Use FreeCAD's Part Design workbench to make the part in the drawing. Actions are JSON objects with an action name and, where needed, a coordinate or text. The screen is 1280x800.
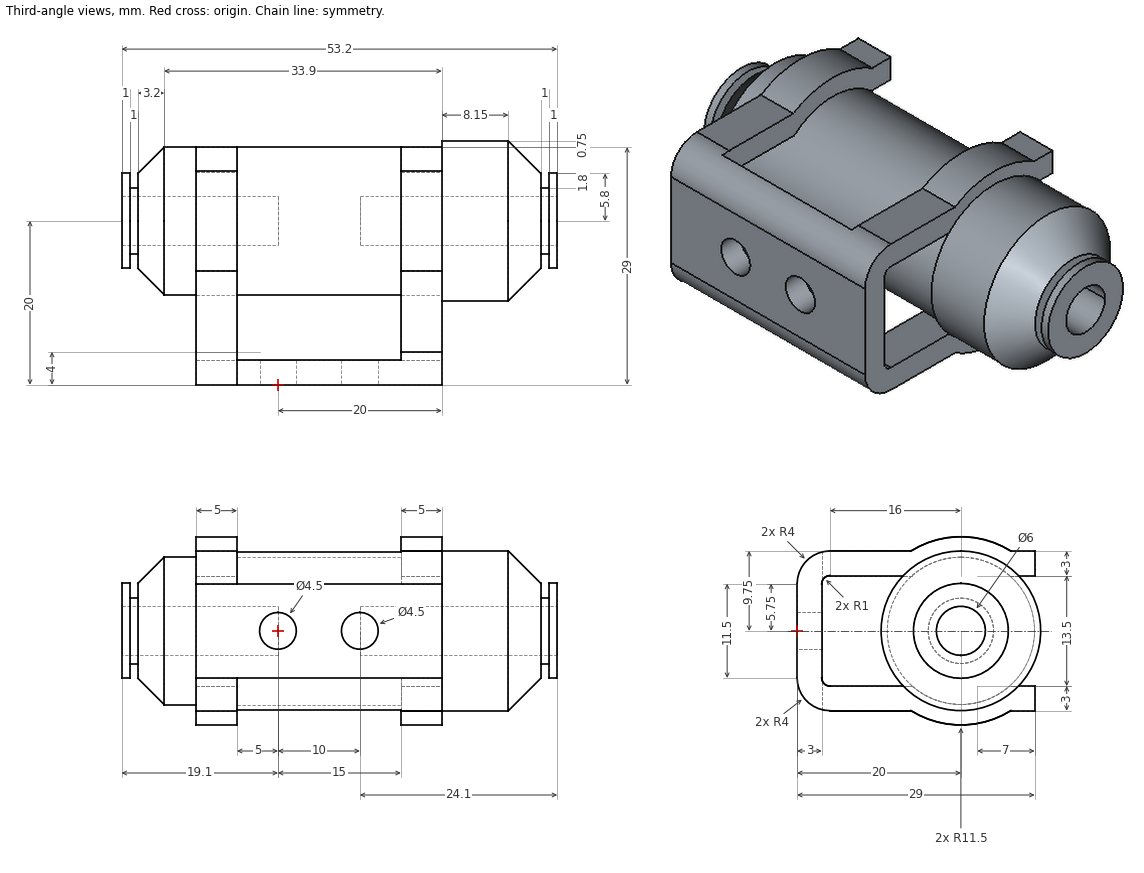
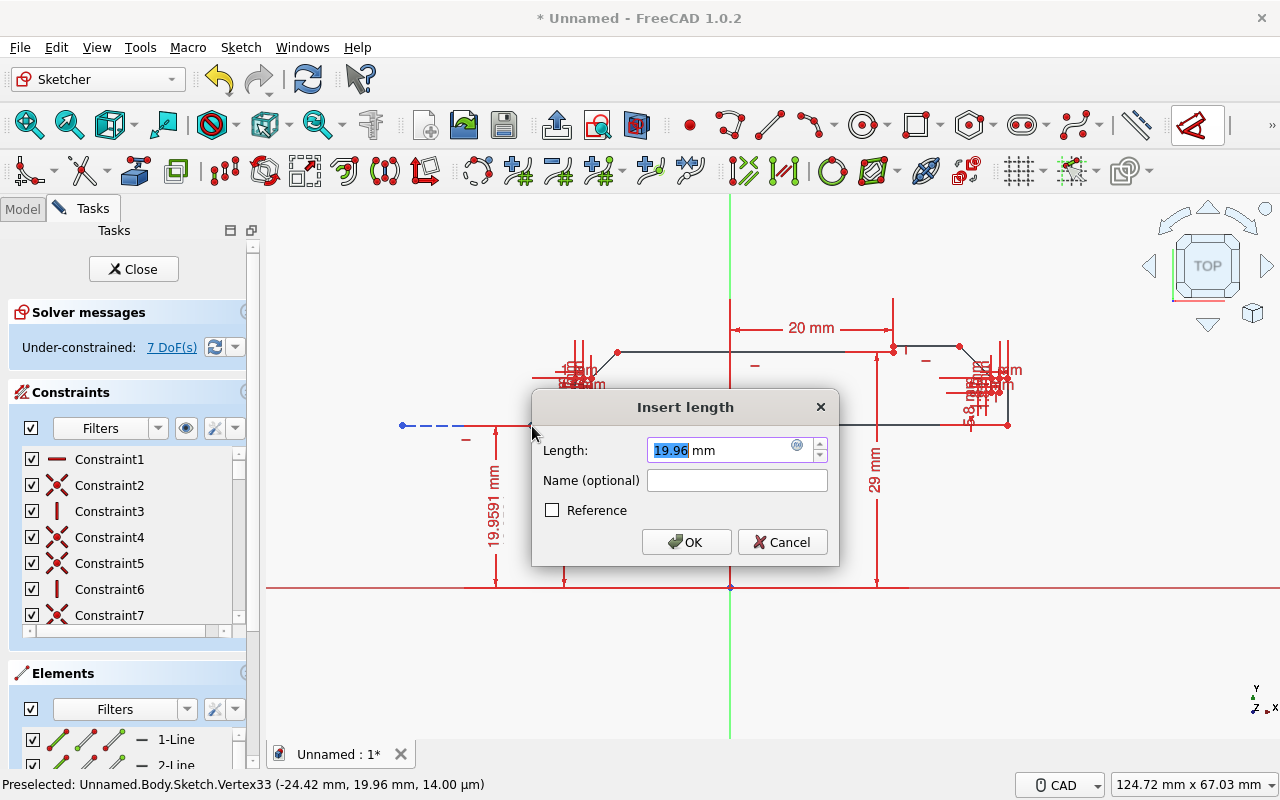
{"action": "type", "text": "20"}
{"action": "key", "text": "Return"}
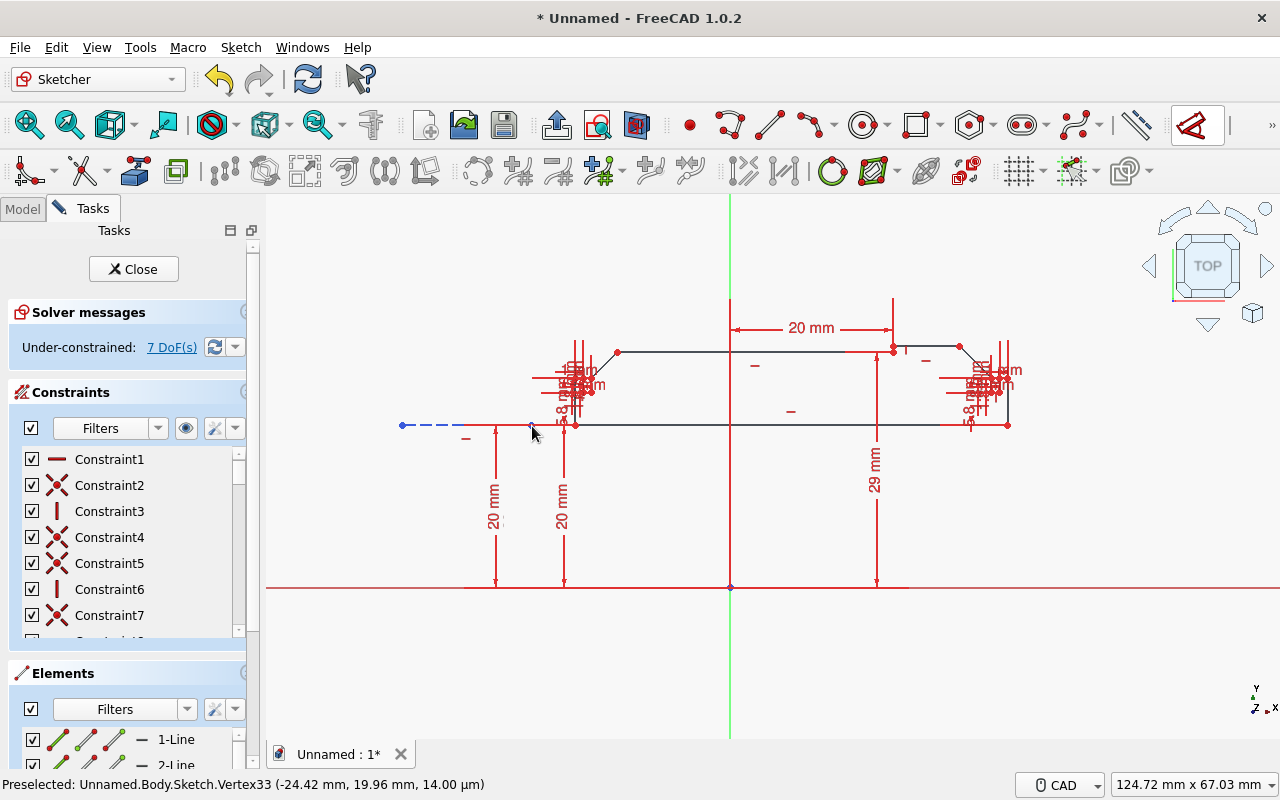
{"action": "left_click", "coordinate": [705, 425]}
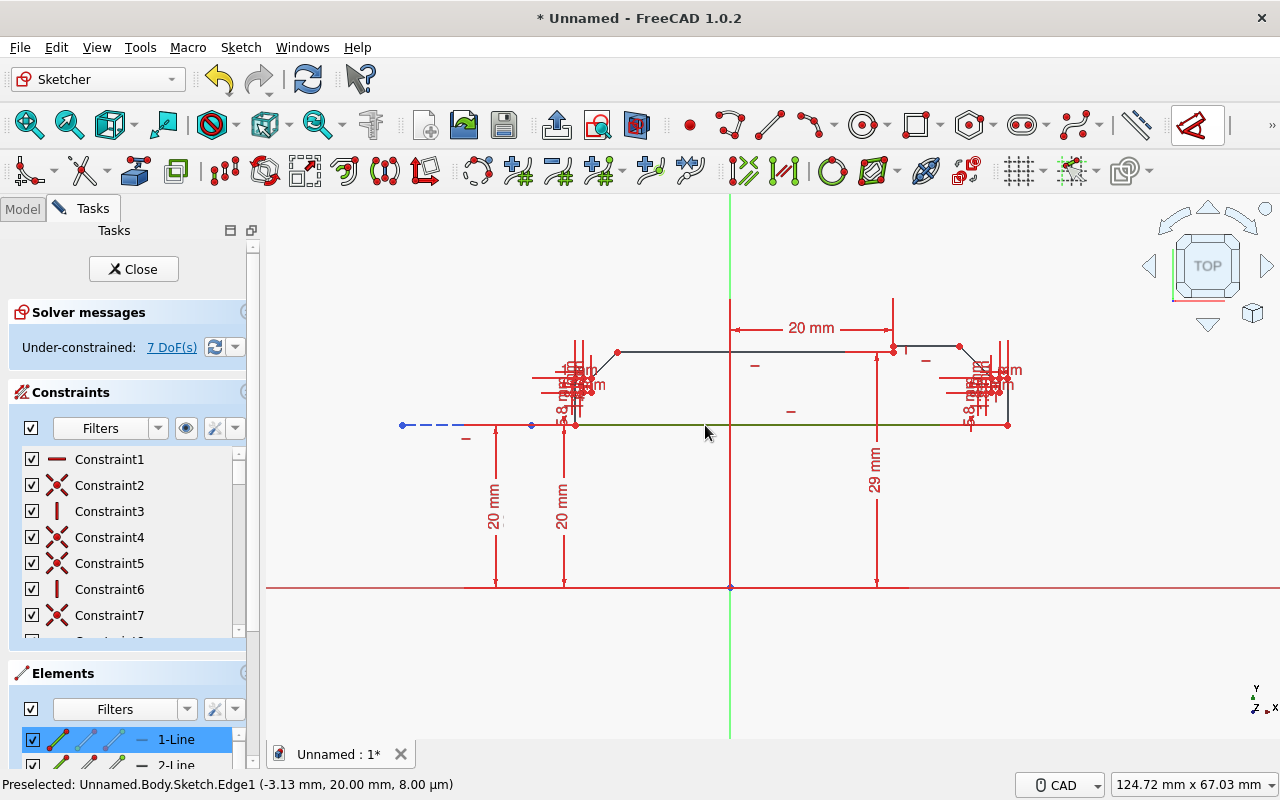
{"action": "left_click", "coordinate": [1218, 126]}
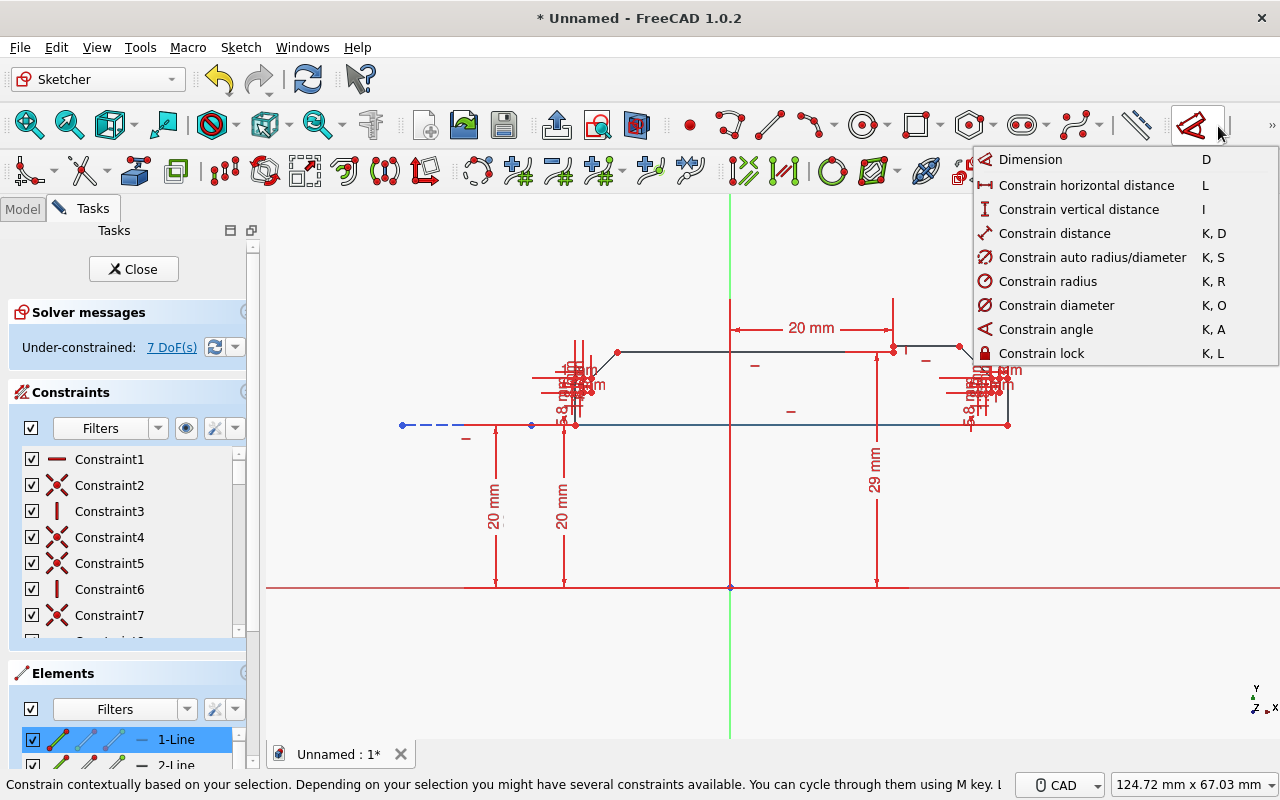
{"action": "left_click", "coordinate": [1126, 185]}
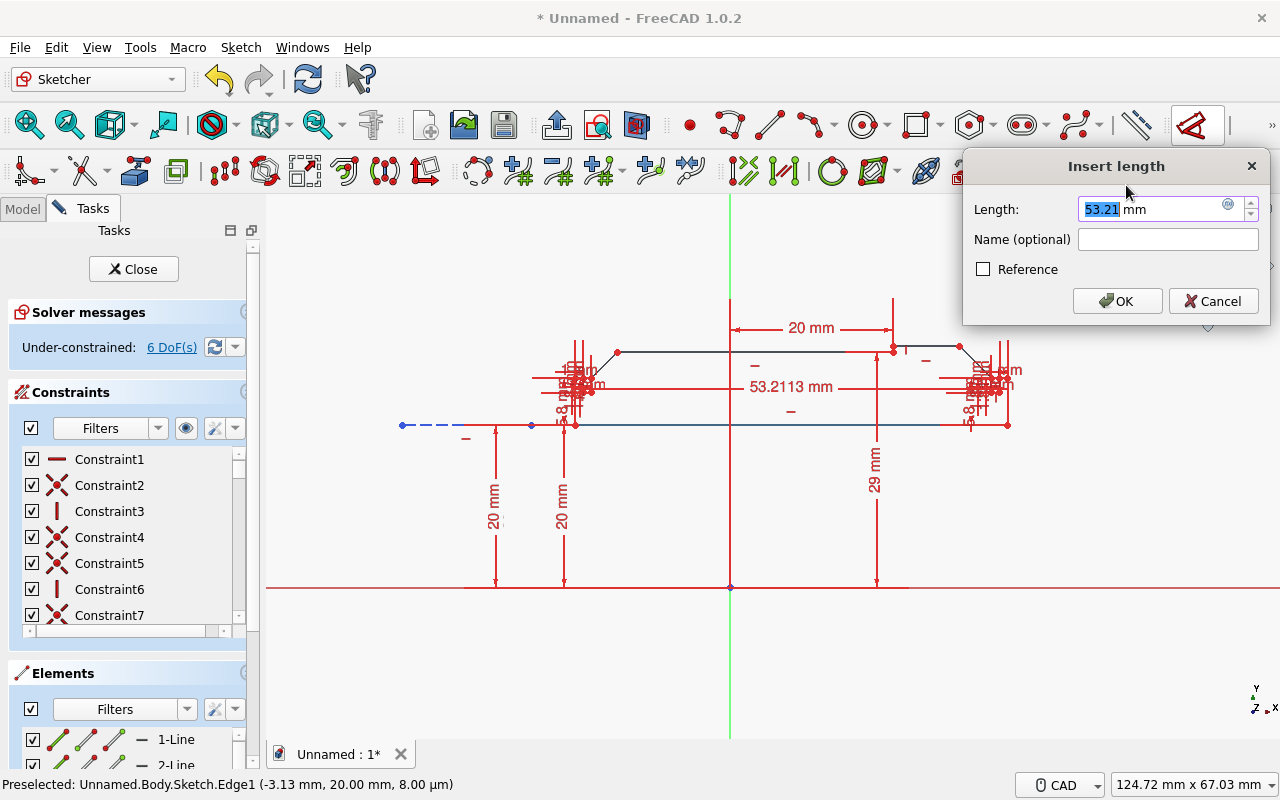
{"action": "type", "text": "53.2"}
{"action": "key", "text": "Return"}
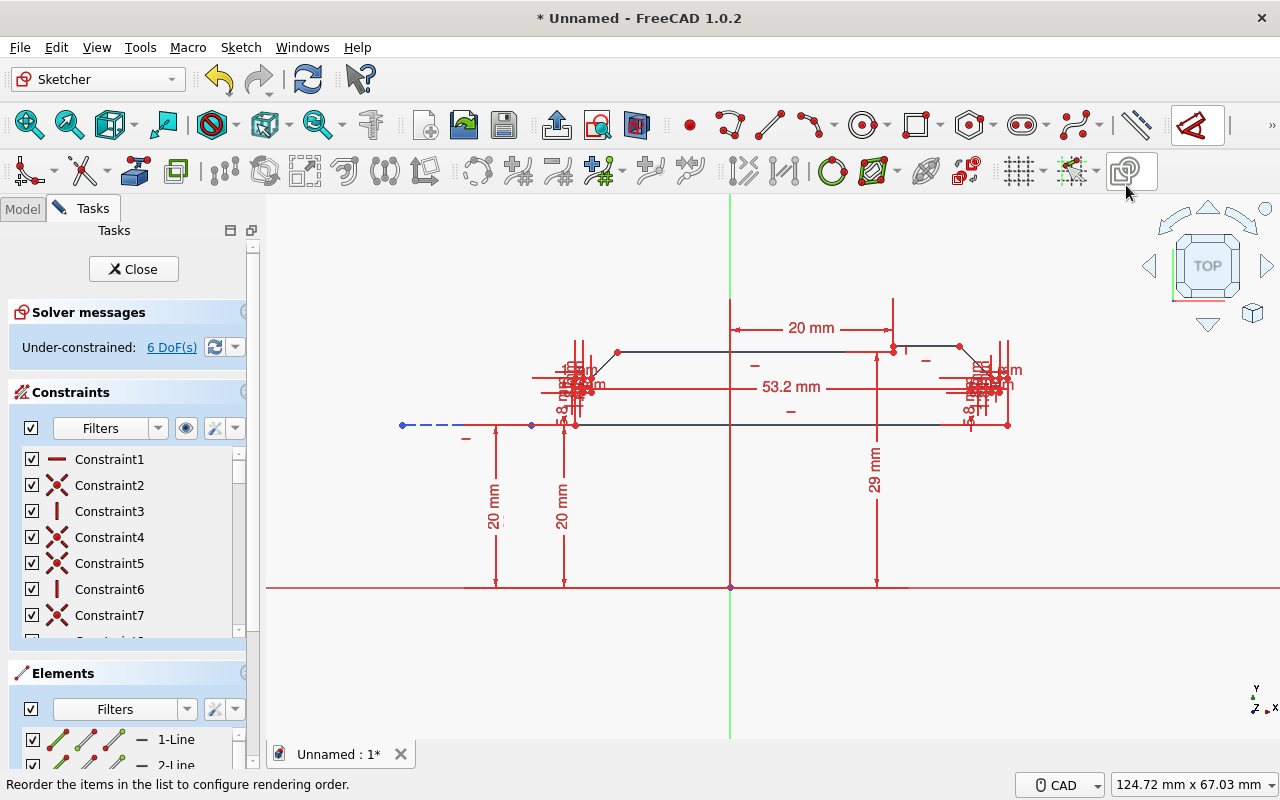
{"action": "left_click", "coordinate": [940, 346]}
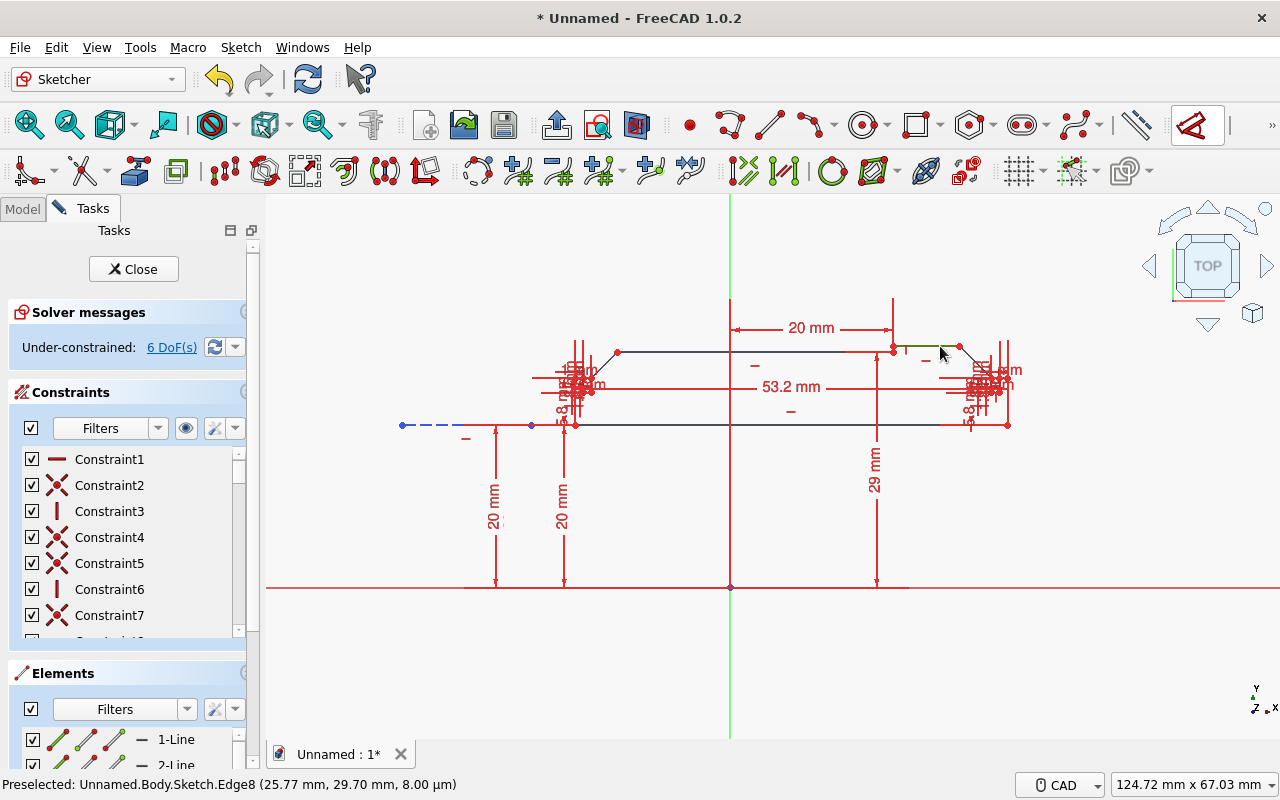
{"action": "key", "text": "l"}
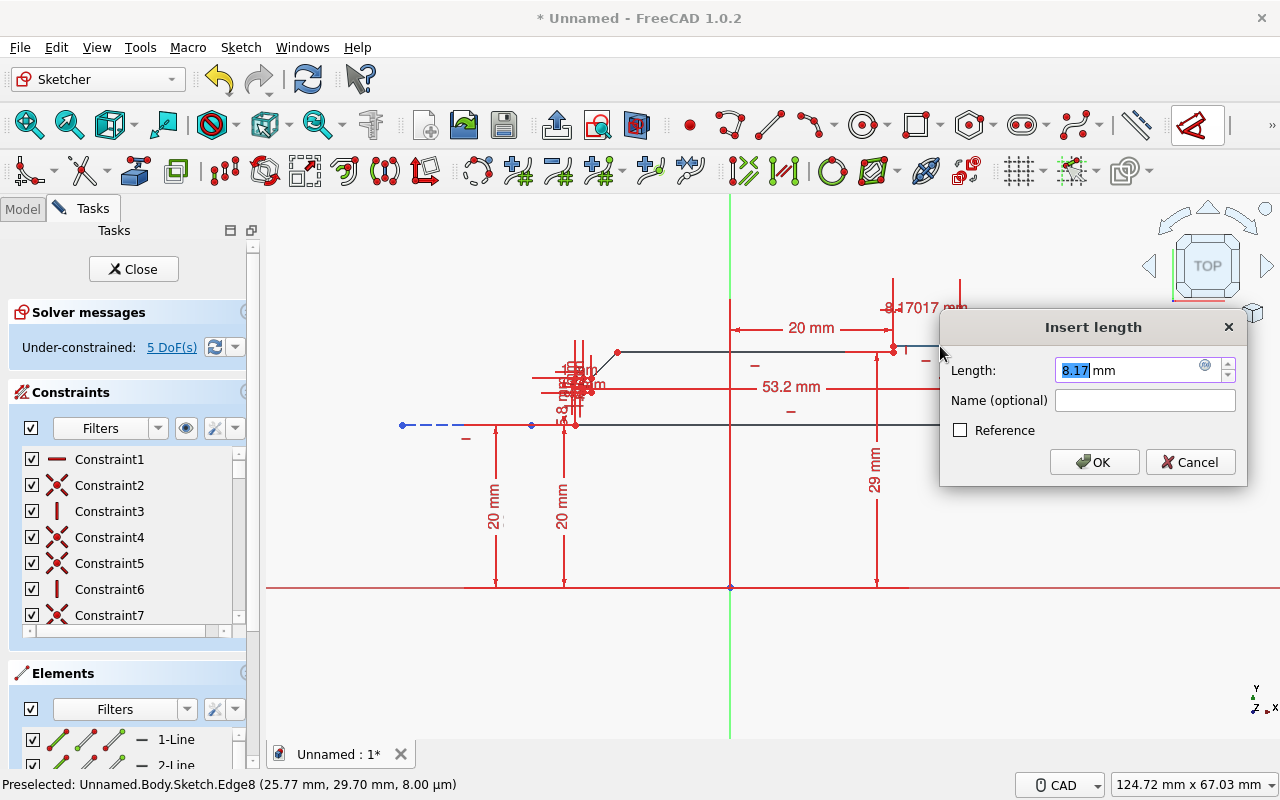
{"action": "type", "text": "8.15"}
{"action": "key", "text": "Return"}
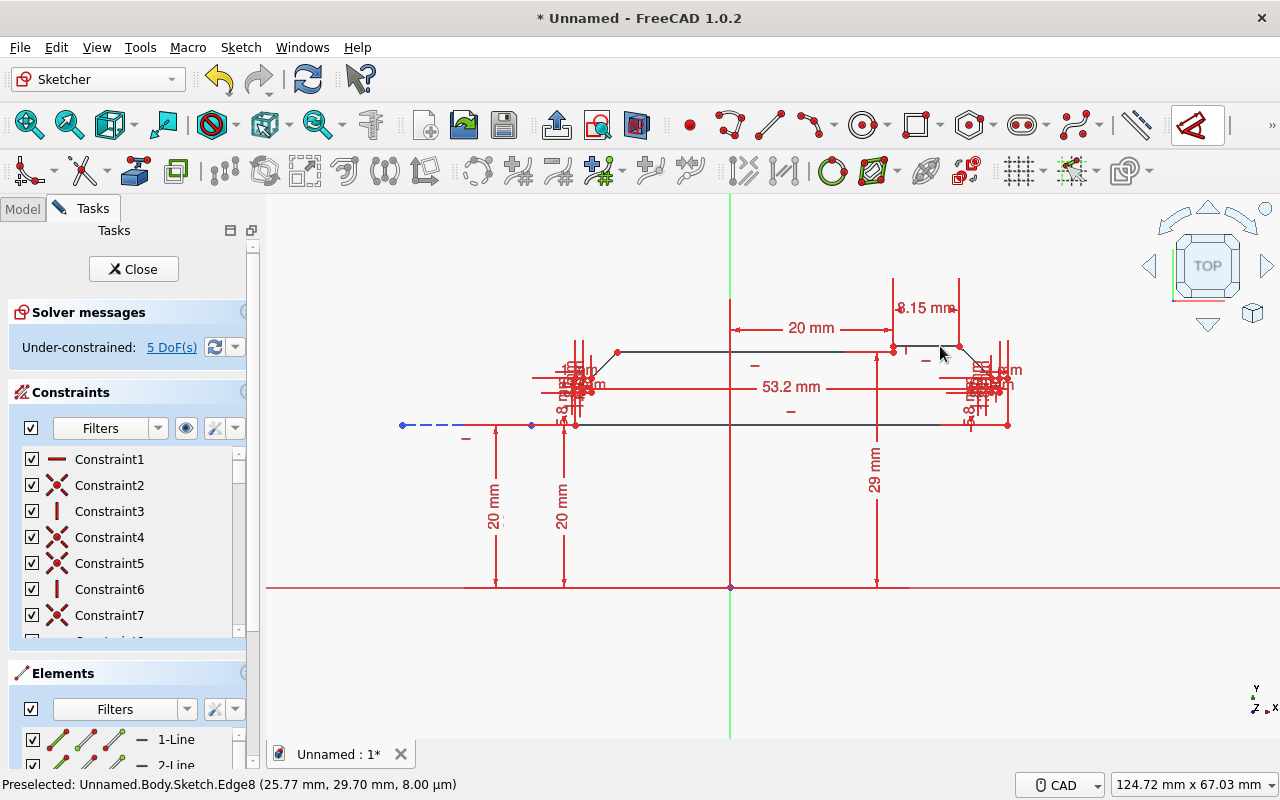
{"action": "scroll", "coordinate": [893, 349], "scroll_direction": "up", "scroll_amount": 10}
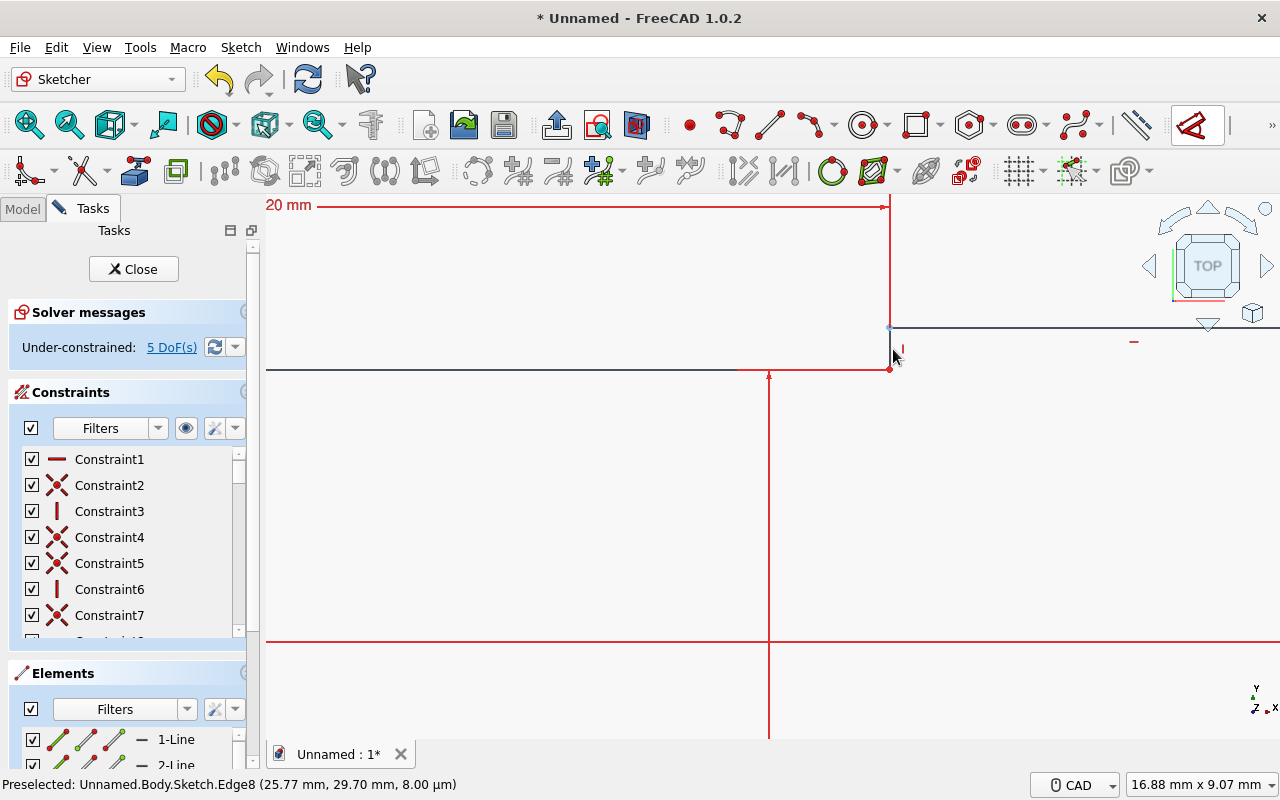
{"action": "left_click", "coordinate": [890, 349]}